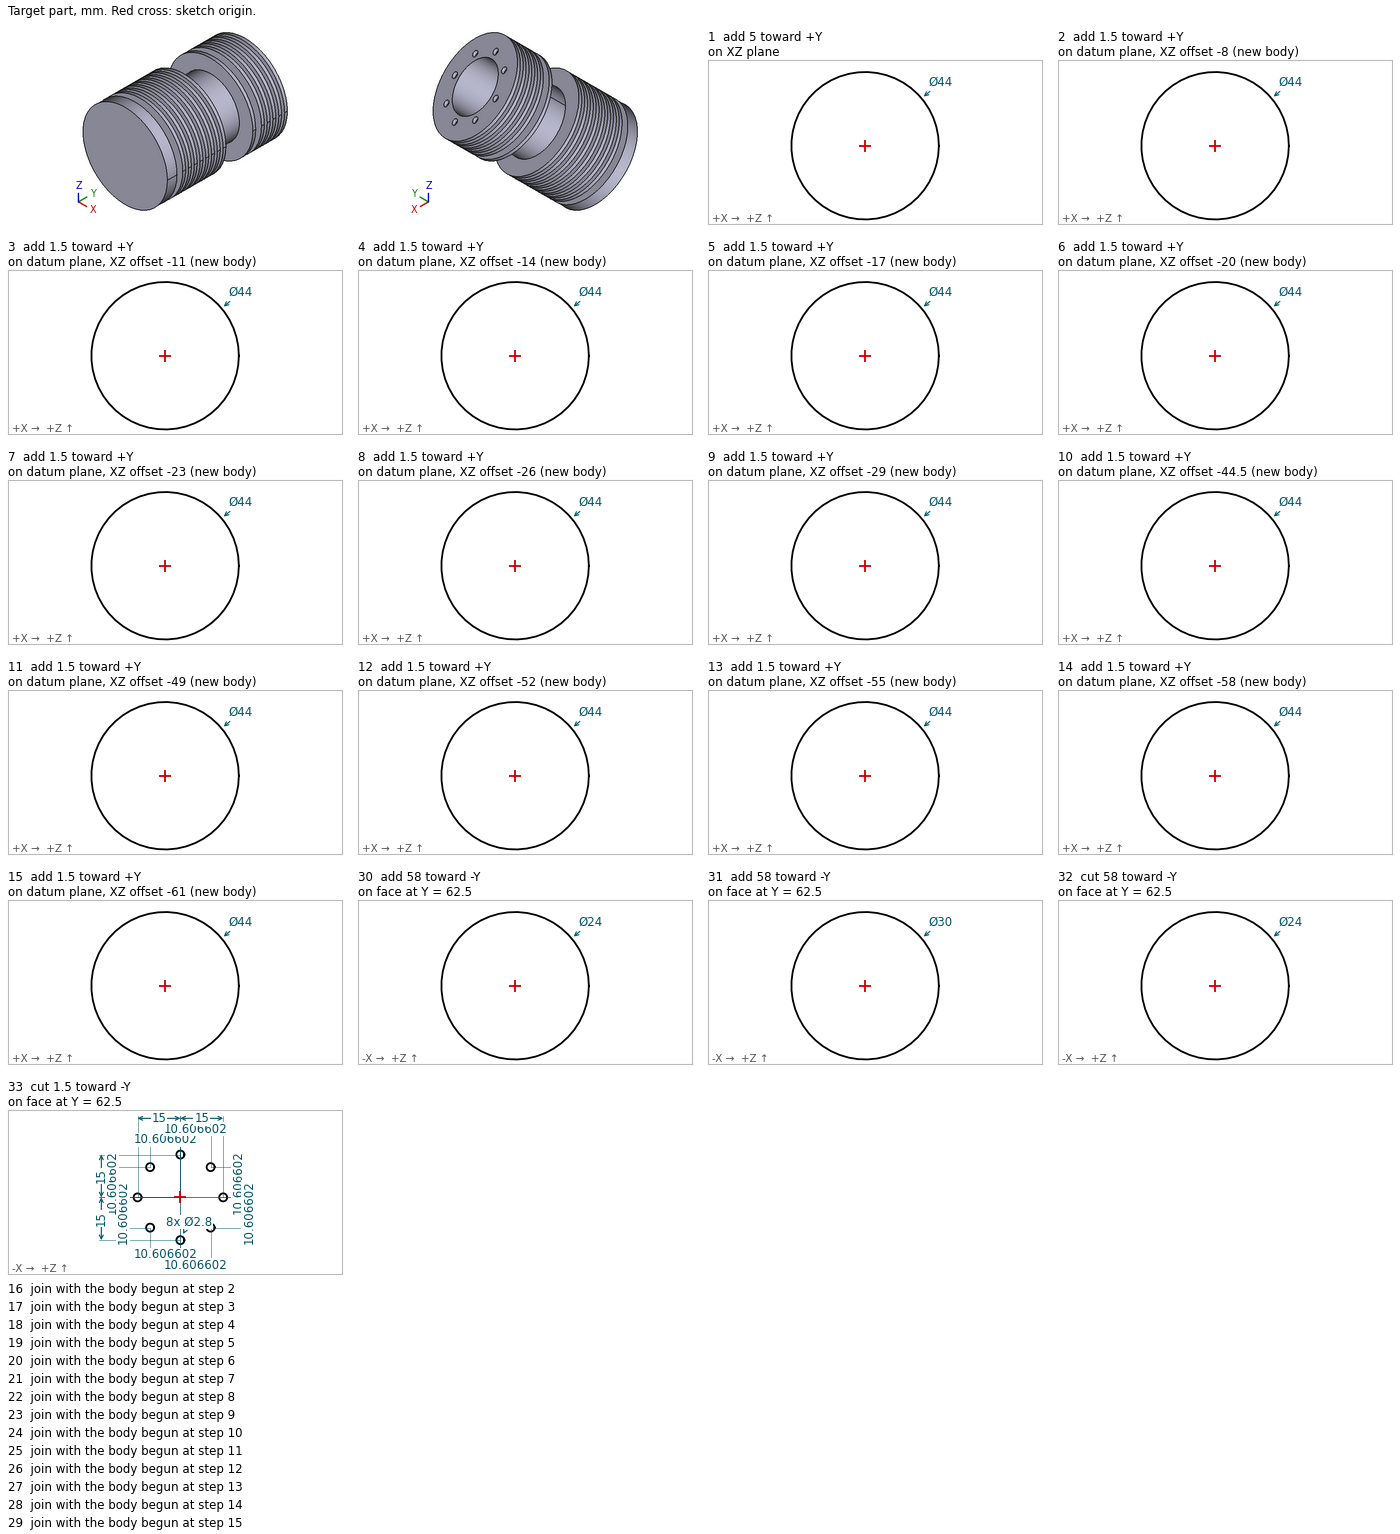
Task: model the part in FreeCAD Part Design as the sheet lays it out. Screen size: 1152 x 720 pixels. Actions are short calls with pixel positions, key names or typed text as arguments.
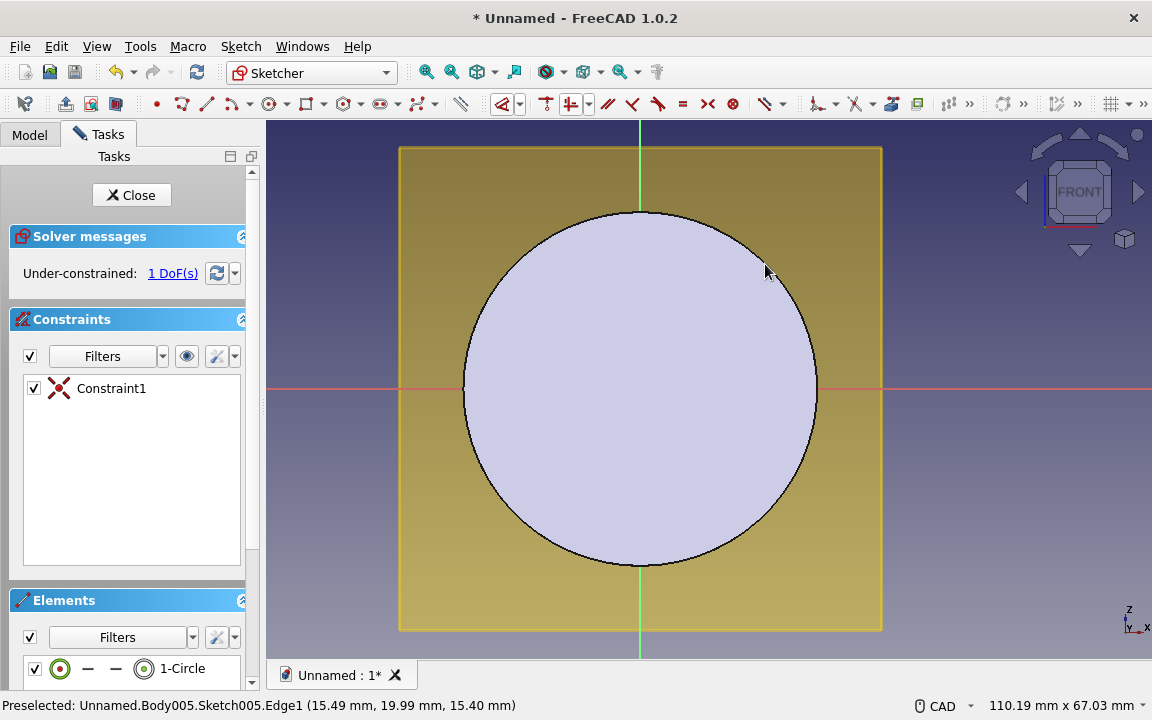
click(764, 264)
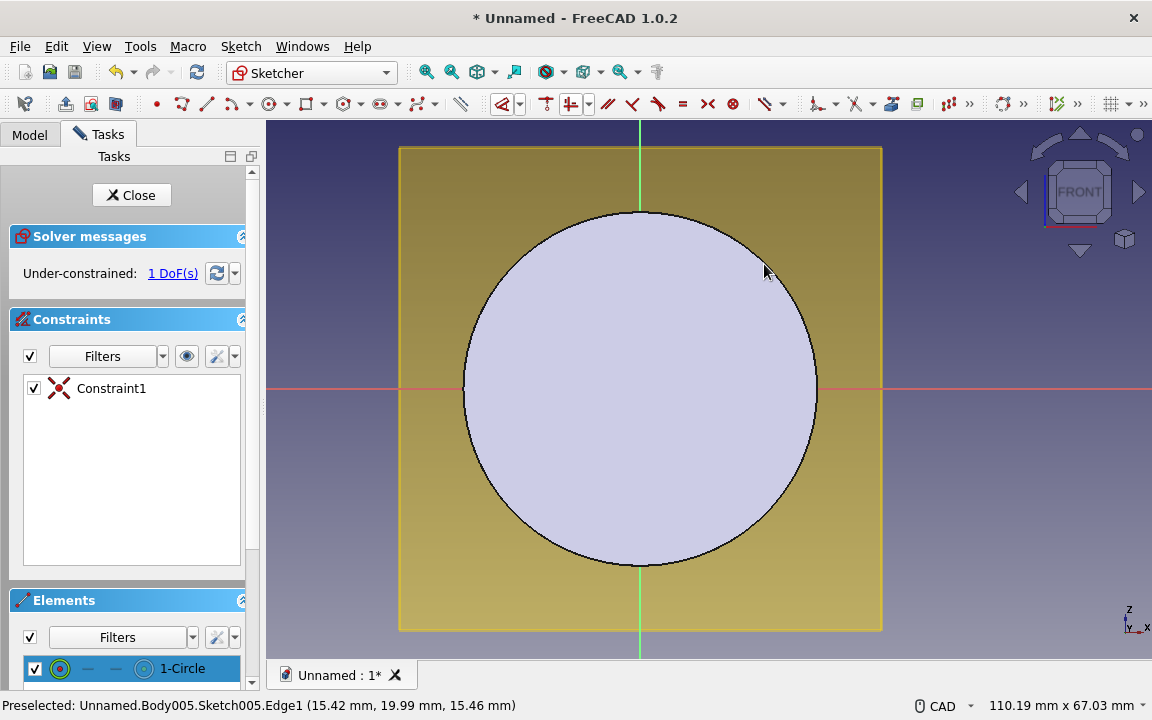
key(k)
key(o)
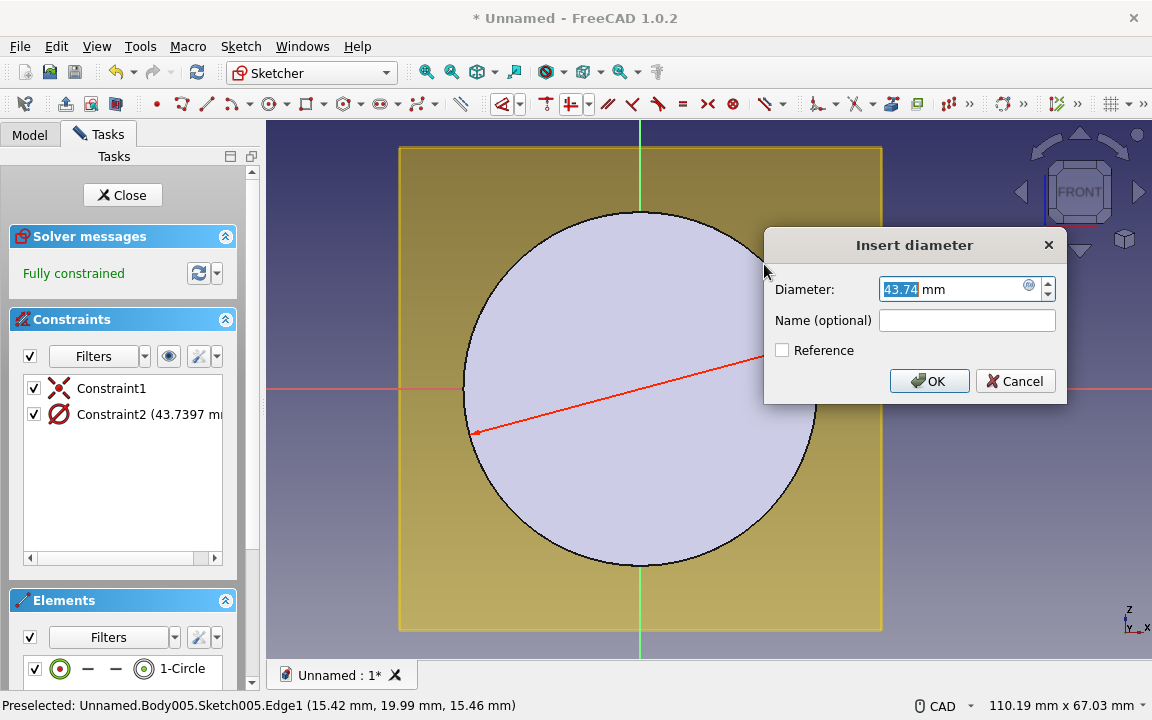
text(44)
key(Return)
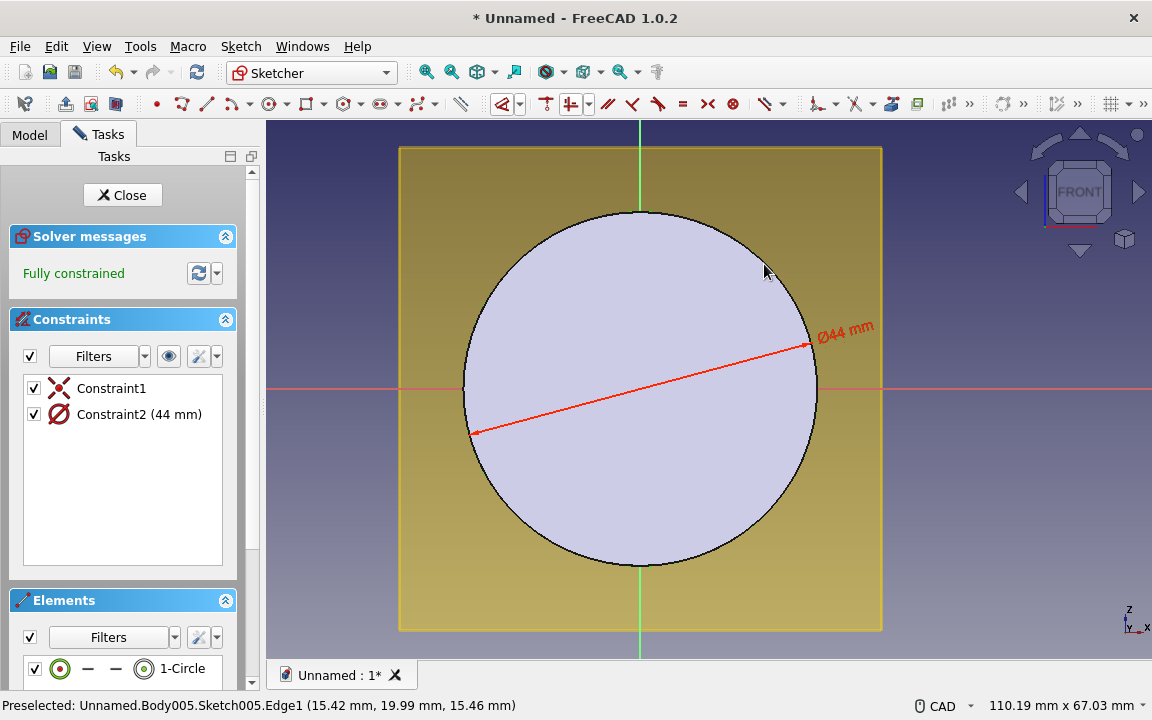
click(123, 195)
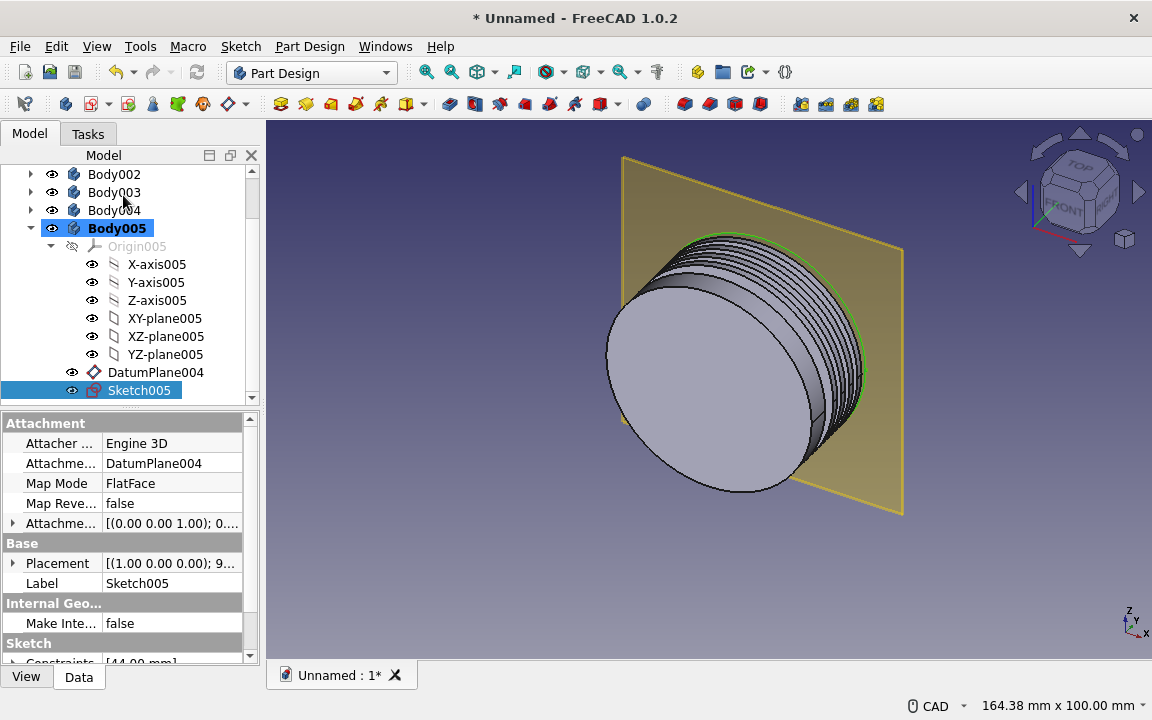
click(281, 104)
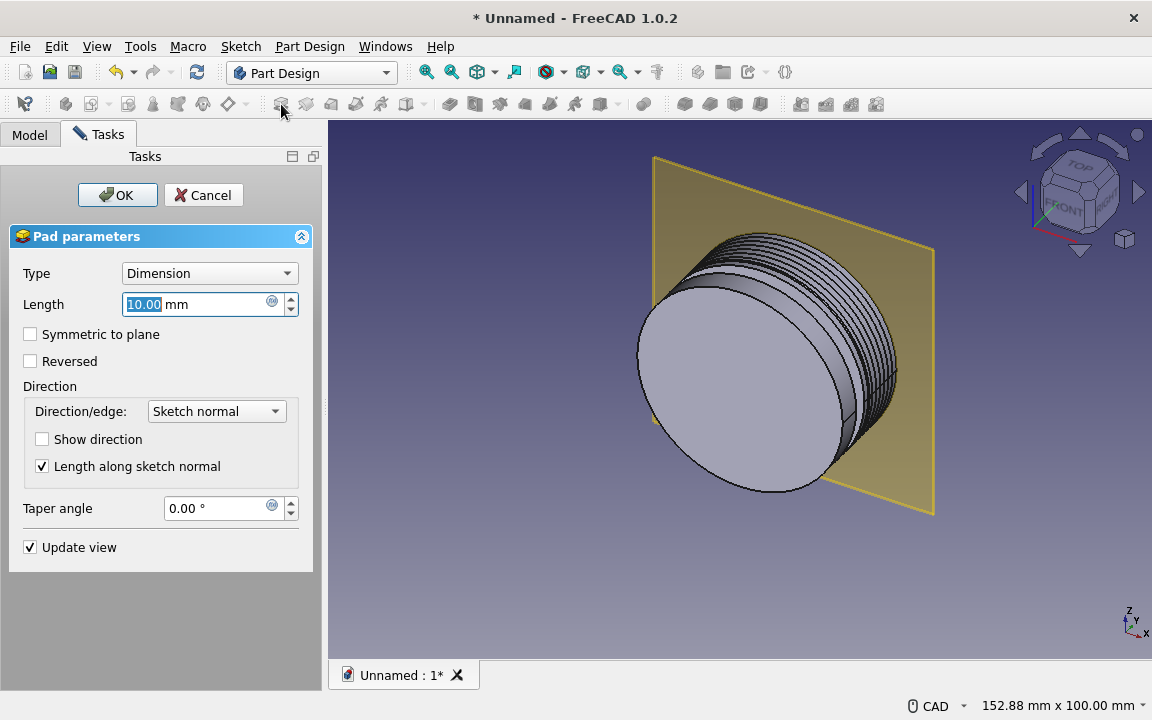
text(1.5)
key(Tab)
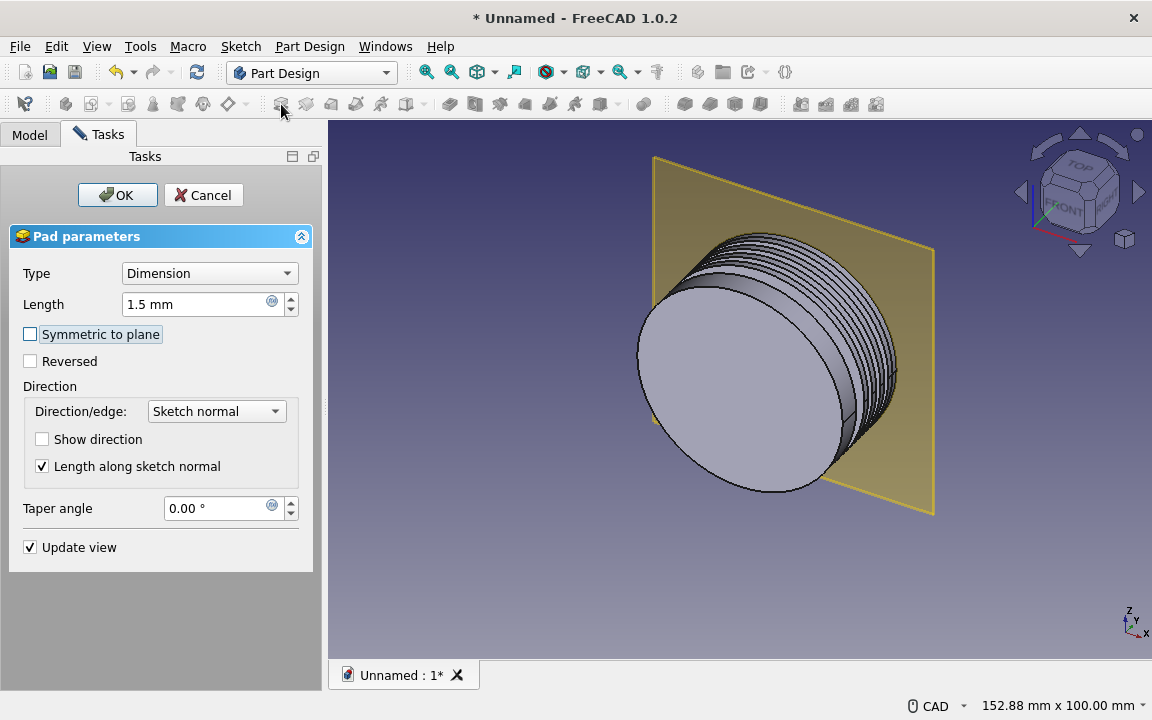
click(31, 361)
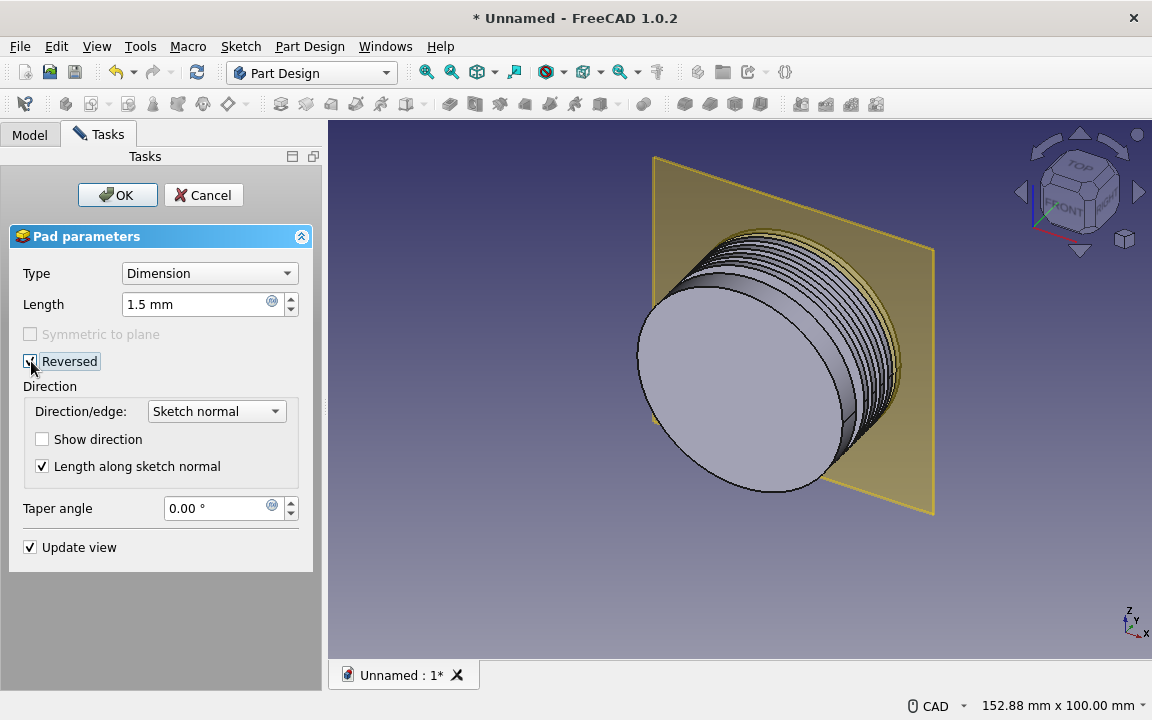
click(118, 195)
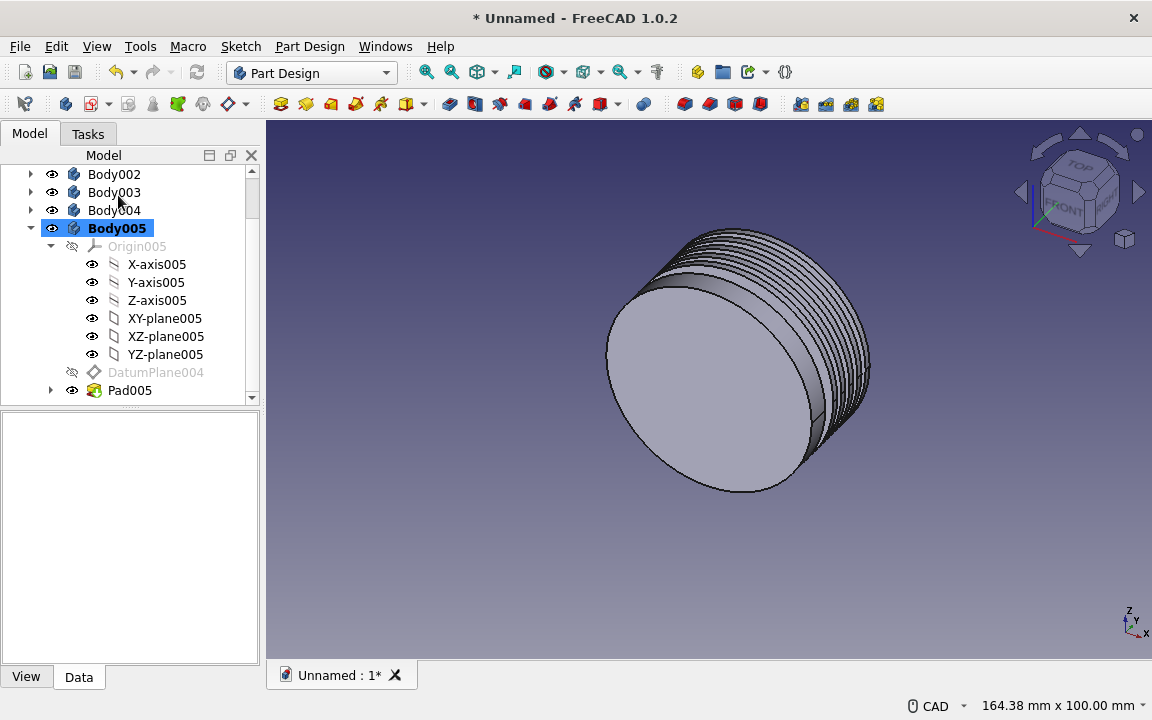
click(66, 104)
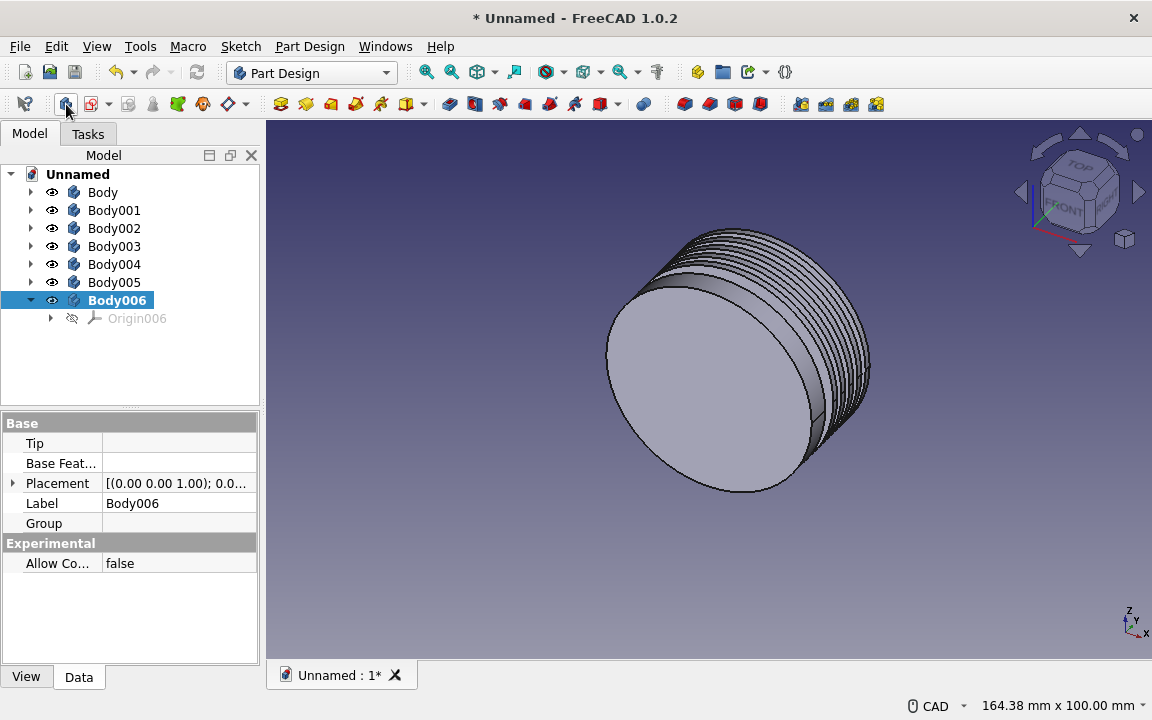
click(51, 318)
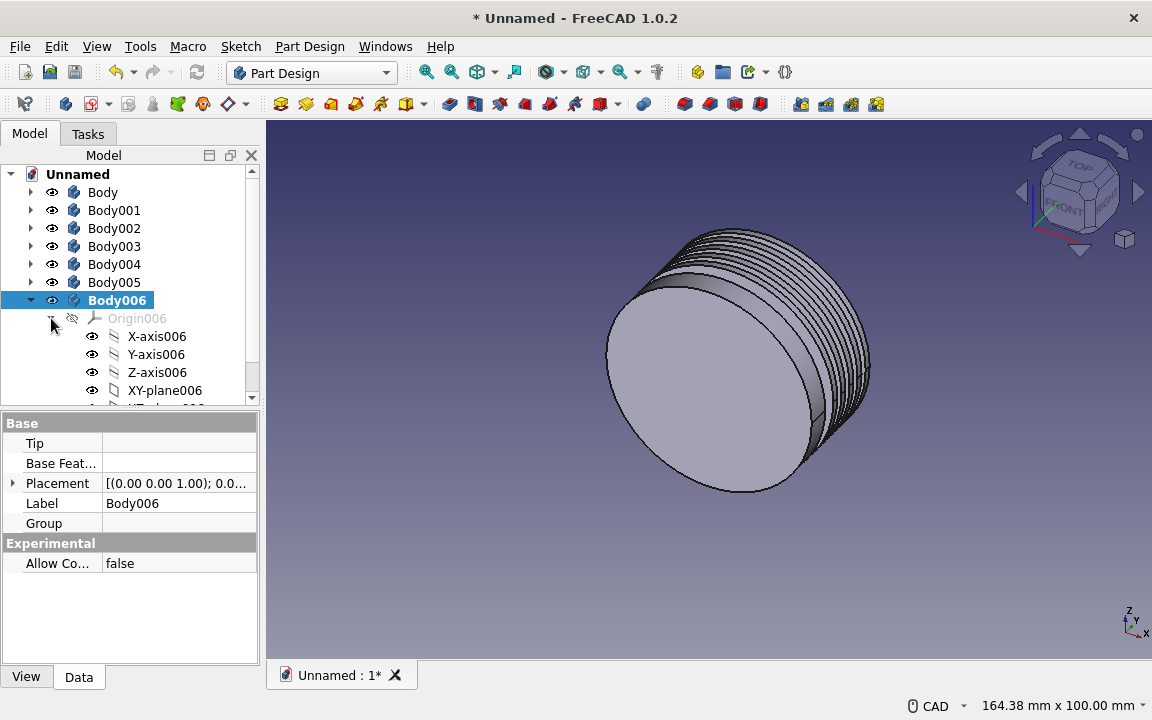
scroll(101, 278, down, 3)